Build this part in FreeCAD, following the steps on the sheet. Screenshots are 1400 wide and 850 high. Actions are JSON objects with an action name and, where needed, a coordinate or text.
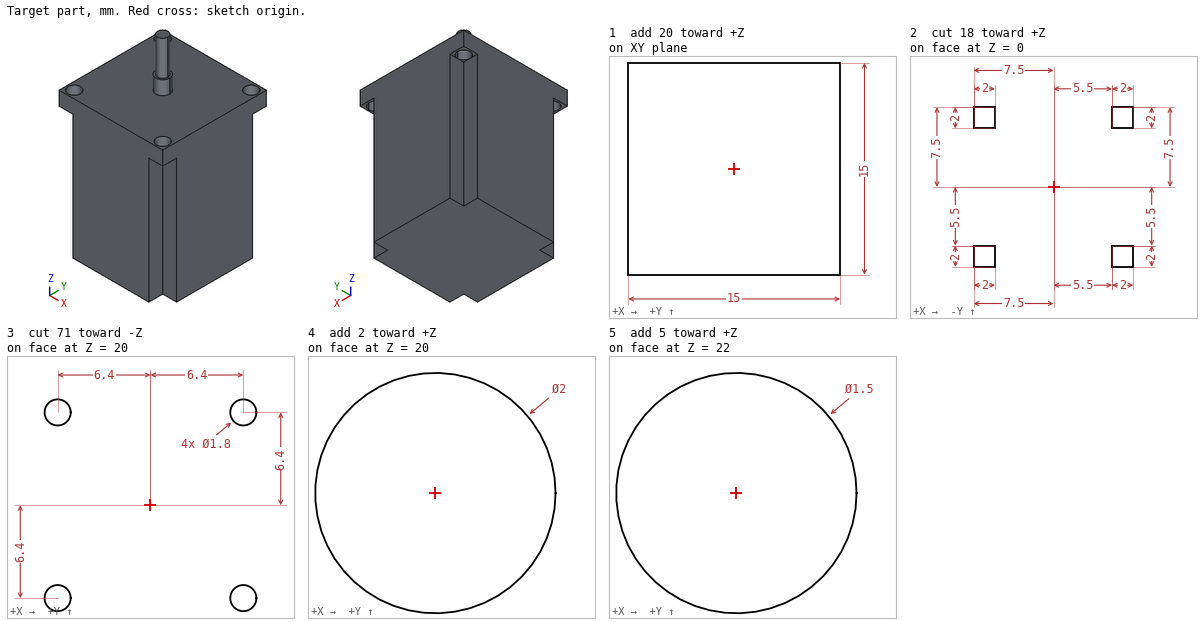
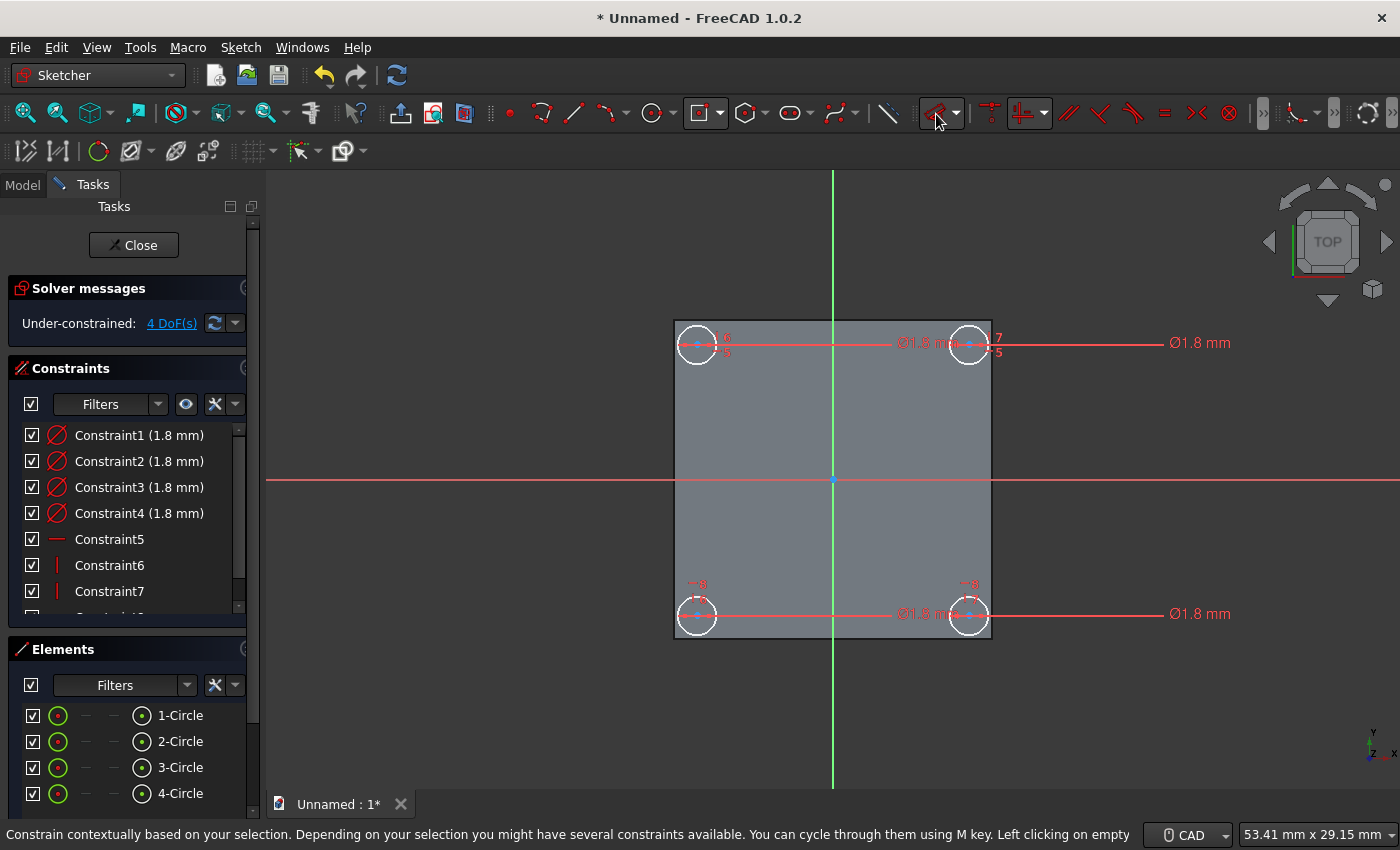
{"action": "left_click", "coordinate": [969, 345]}
{"action": "left_click", "coordinate": [901, 311]}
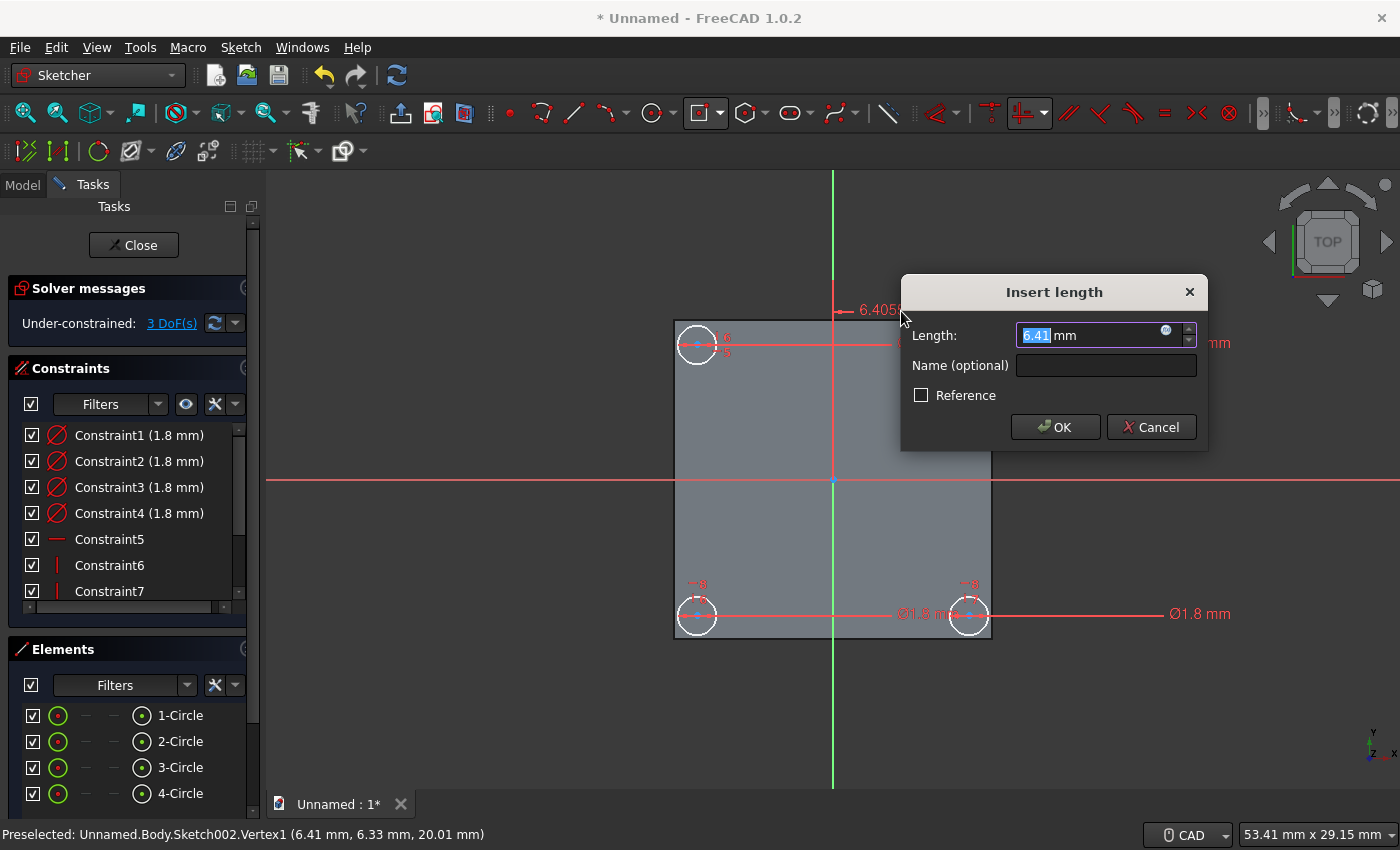
{"action": "type", "text": "6.4"}
{"action": "key", "text": "Return"}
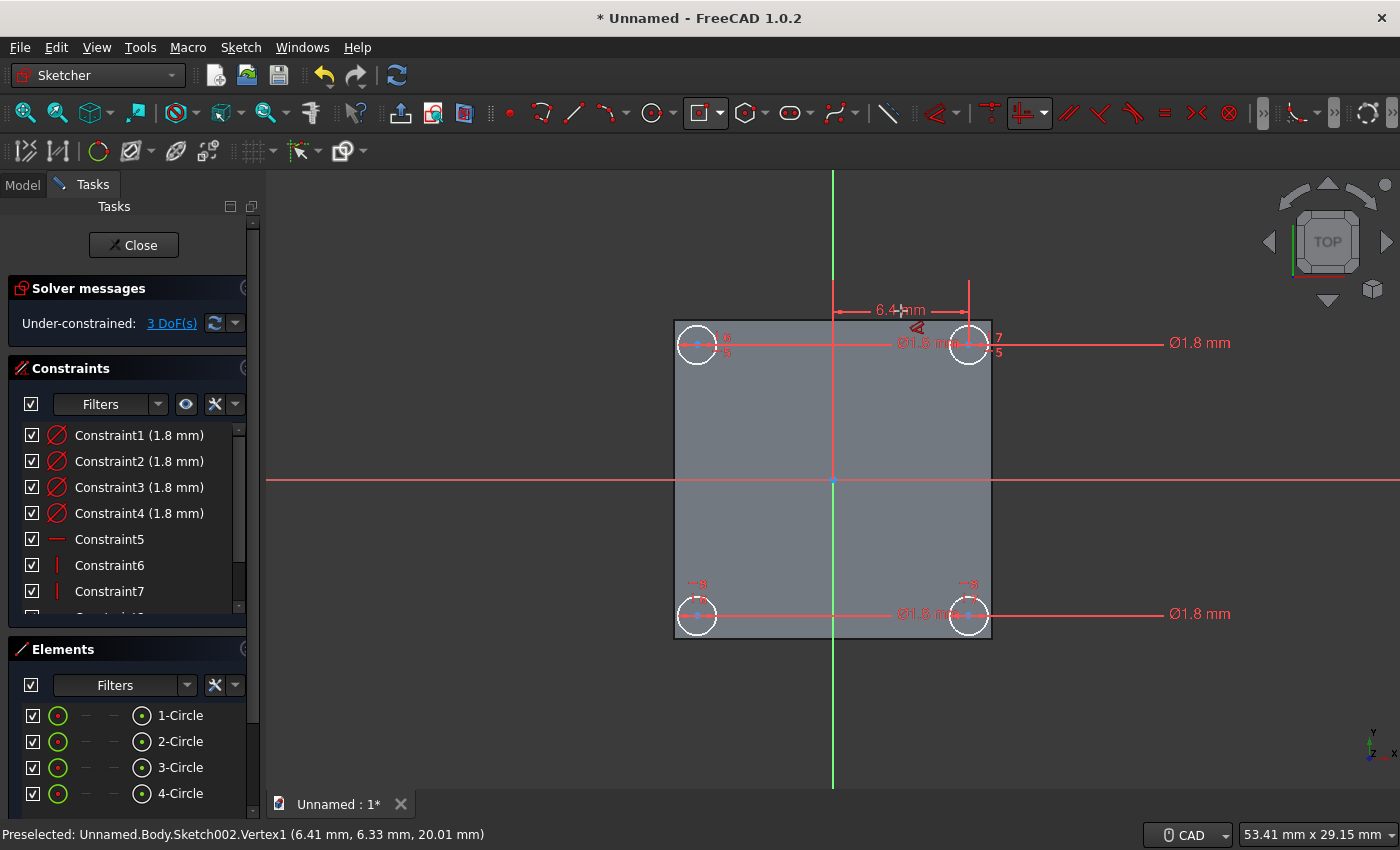
{"action": "left_click", "coordinate": [969, 345]}
{"action": "left_click", "coordinate": [1003, 412]}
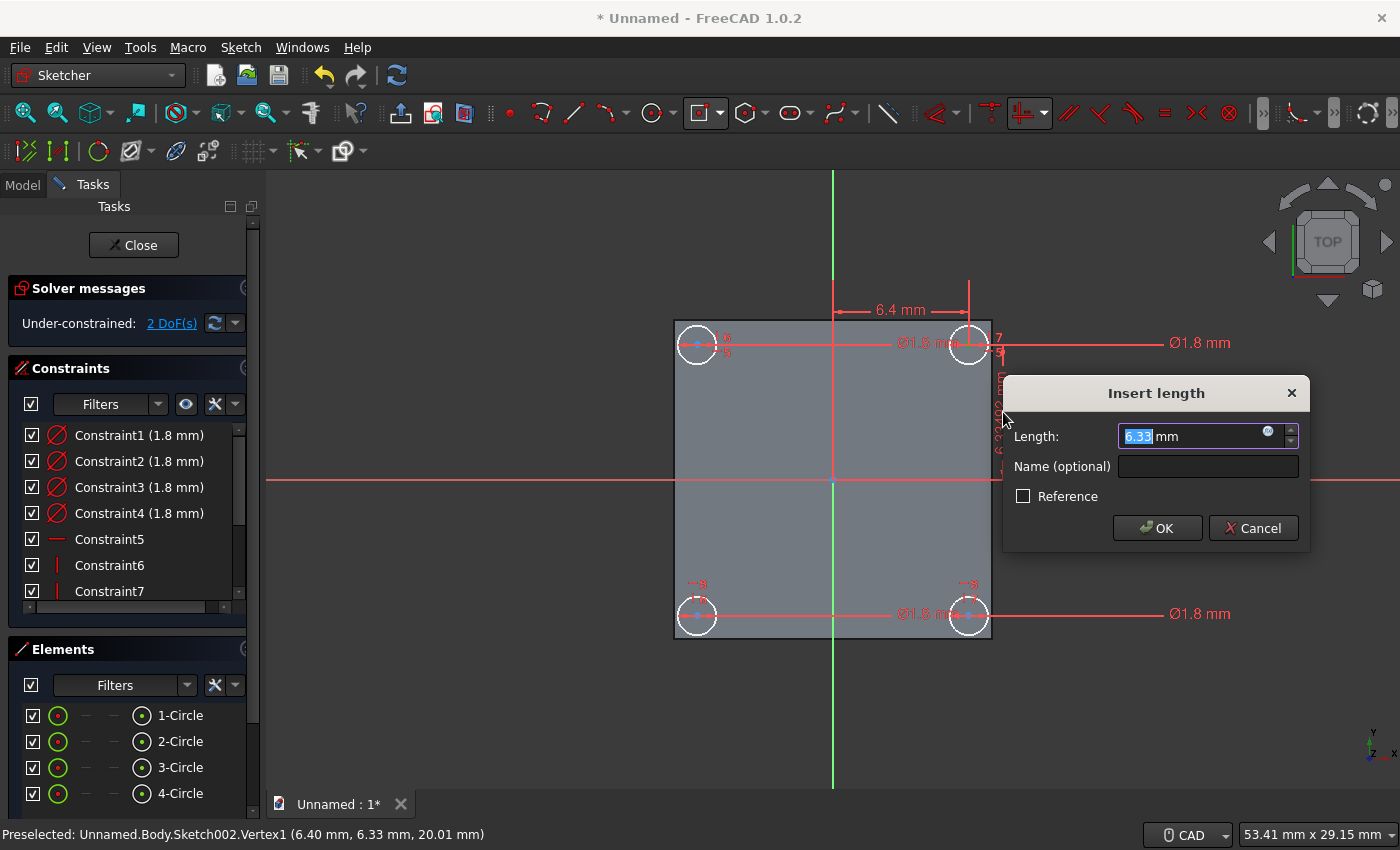
{"action": "type", "text": "6.4"}
{"action": "key", "text": "Return"}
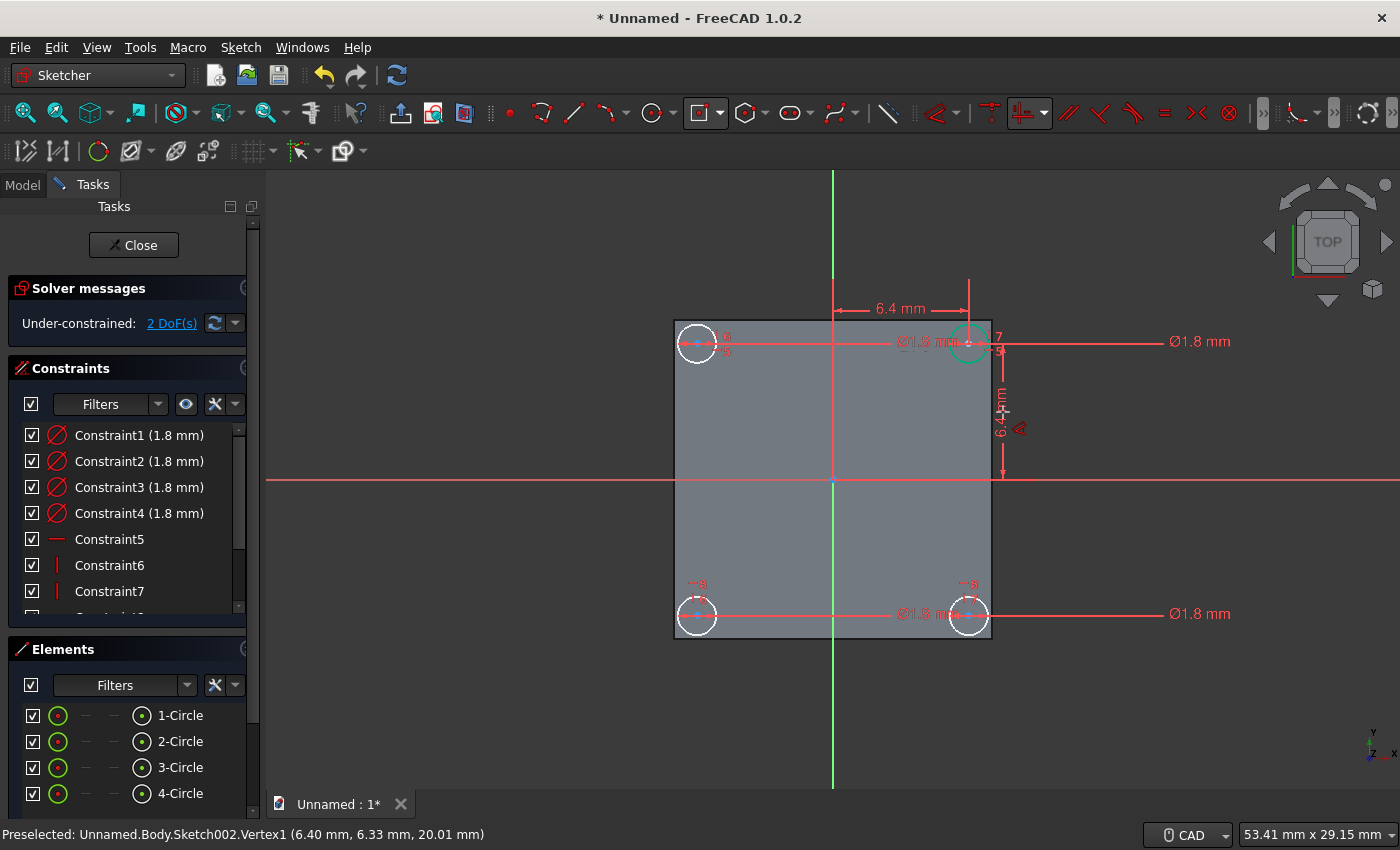
{"action": "left_click", "coordinate": [697, 344]}
{"action": "left_click", "coordinate": [765, 310]}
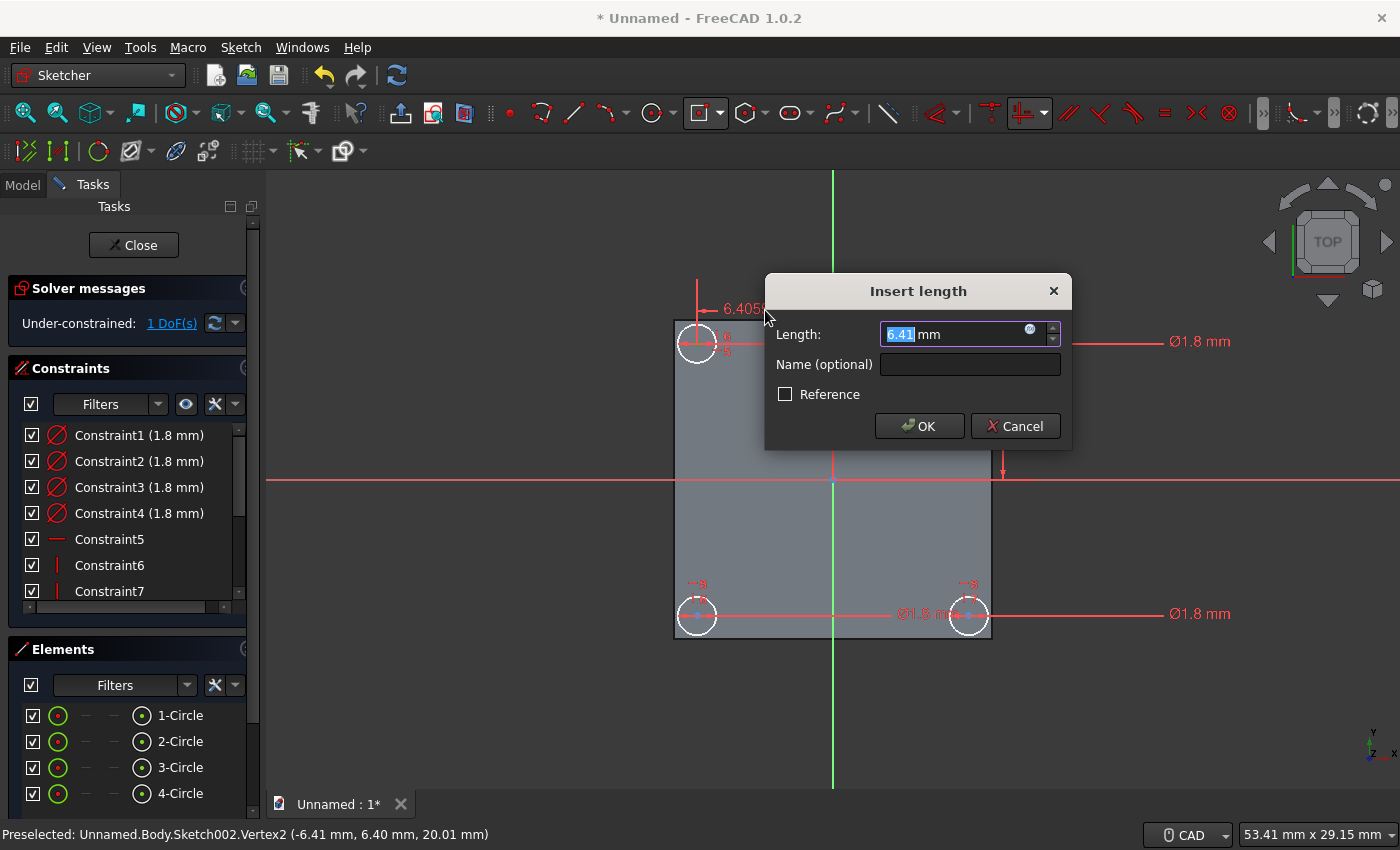
{"action": "type", "text": "6.4"}
{"action": "key", "text": "Return"}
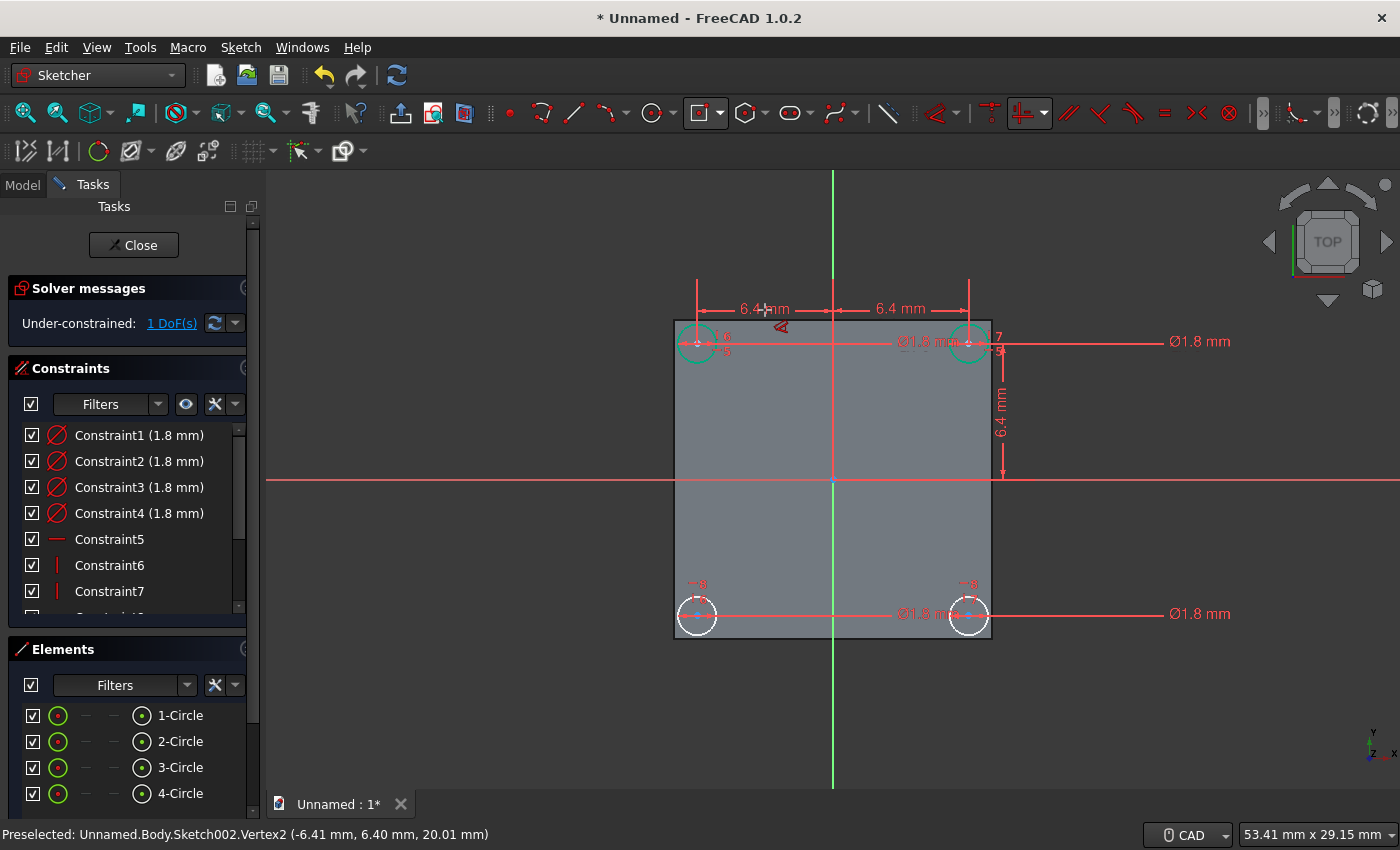
{"action": "left_click", "coordinate": [697, 616]}
{"action": "left_click", "coordinate": [663, 548]}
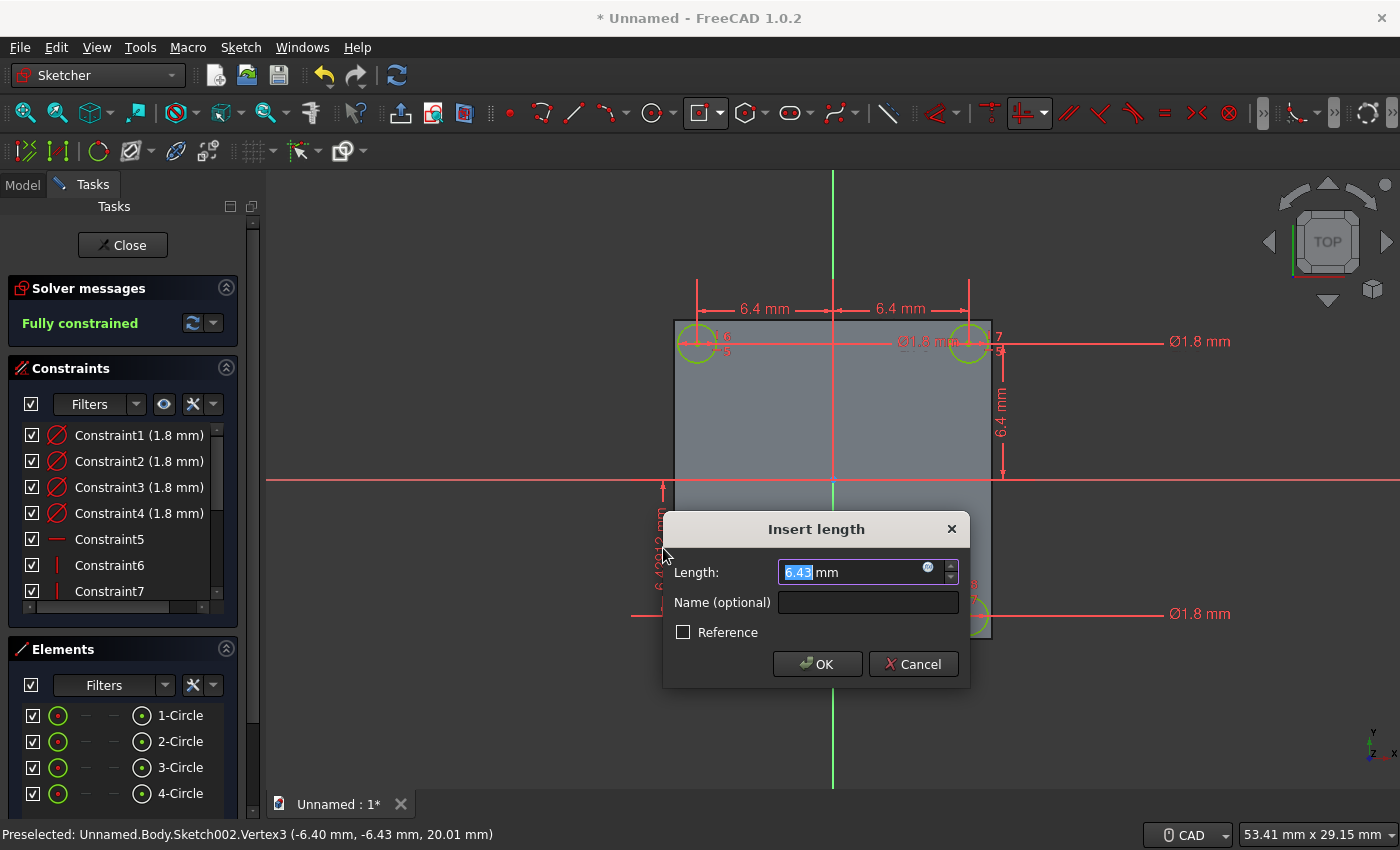
{"action": "type", "text": "6.4"}
{"action": "key", "text": "Return"}
{"action": "key", "text": "Escape"}